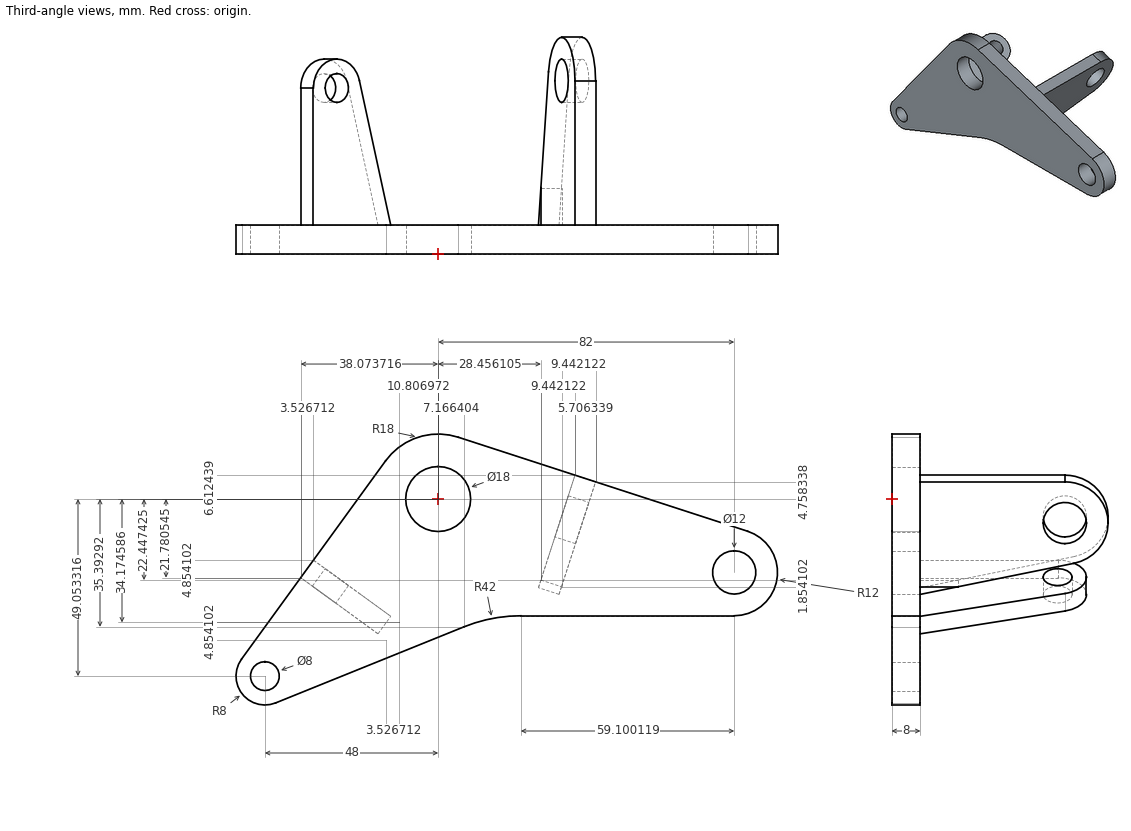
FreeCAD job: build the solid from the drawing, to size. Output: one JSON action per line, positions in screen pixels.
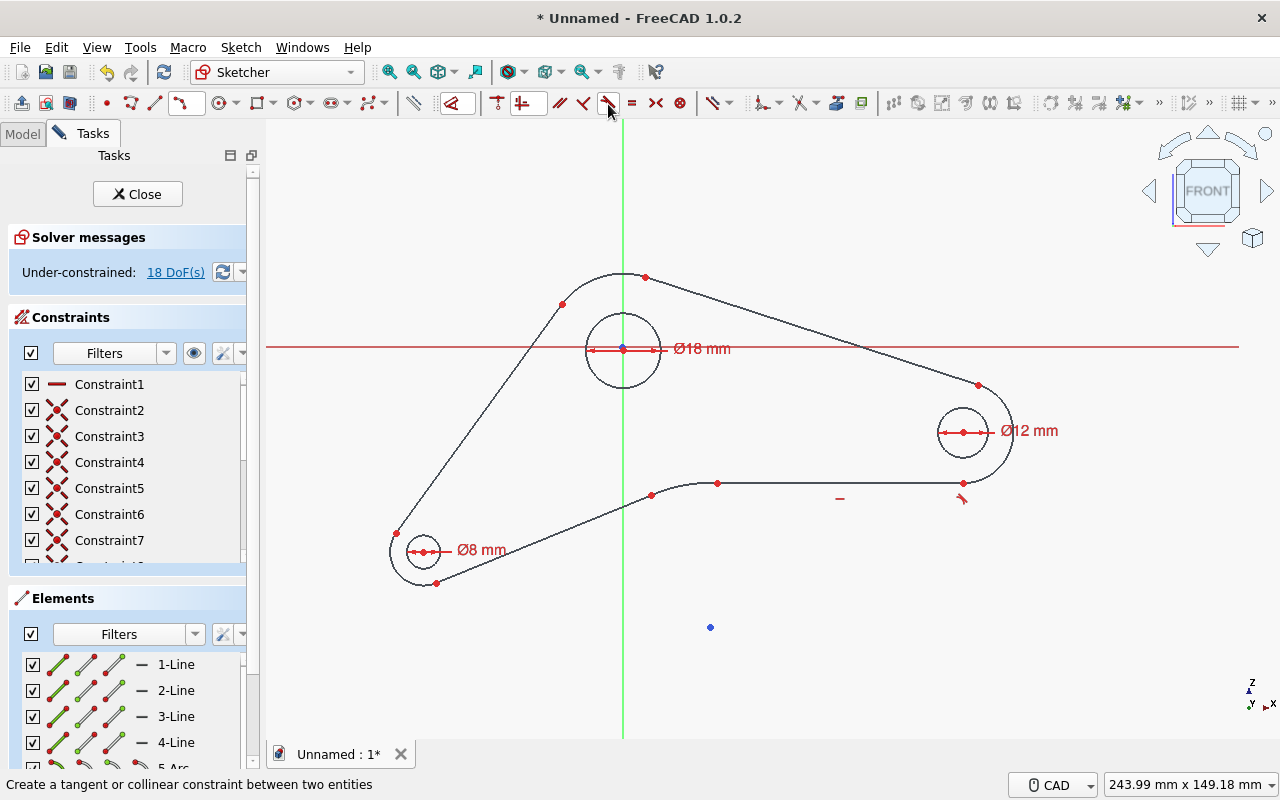
{"action": "left_click", "coordinate": [587, 522]}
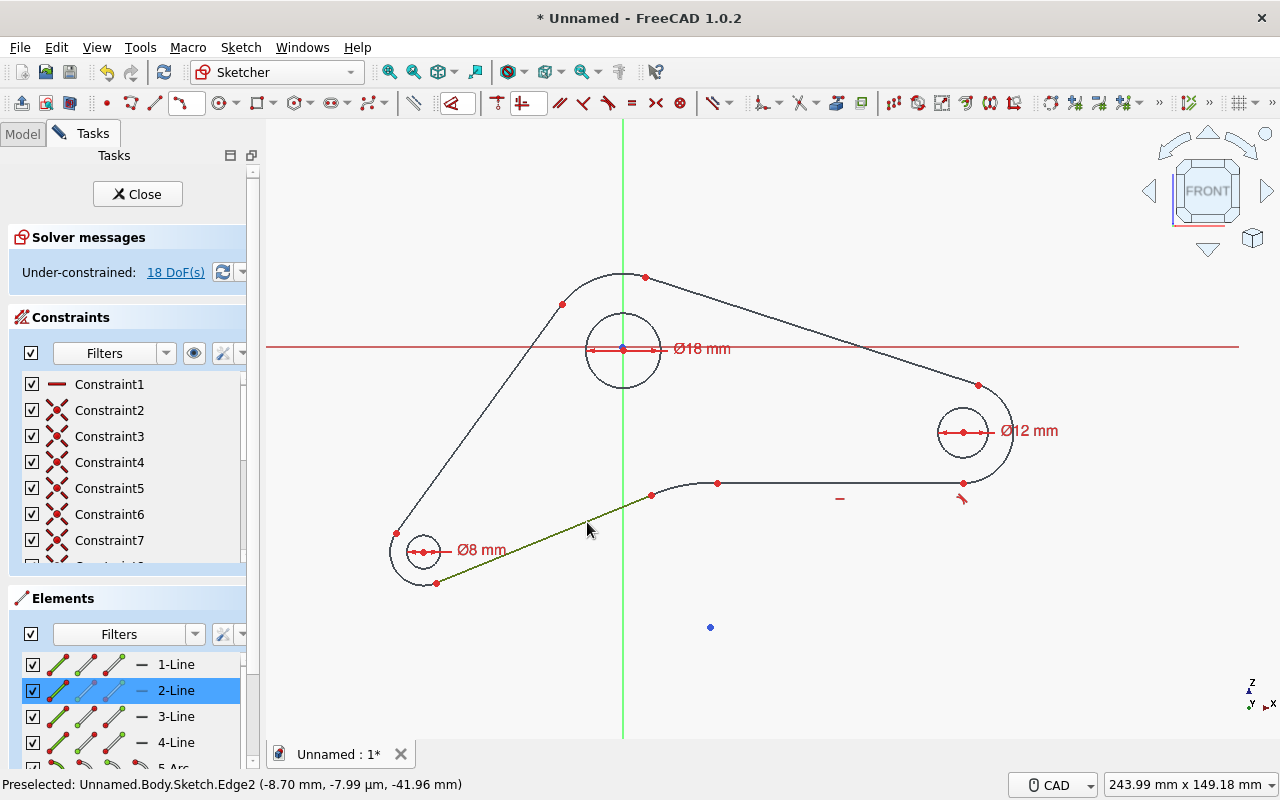
{"action": "left_click", "coordinate": [698, 483]}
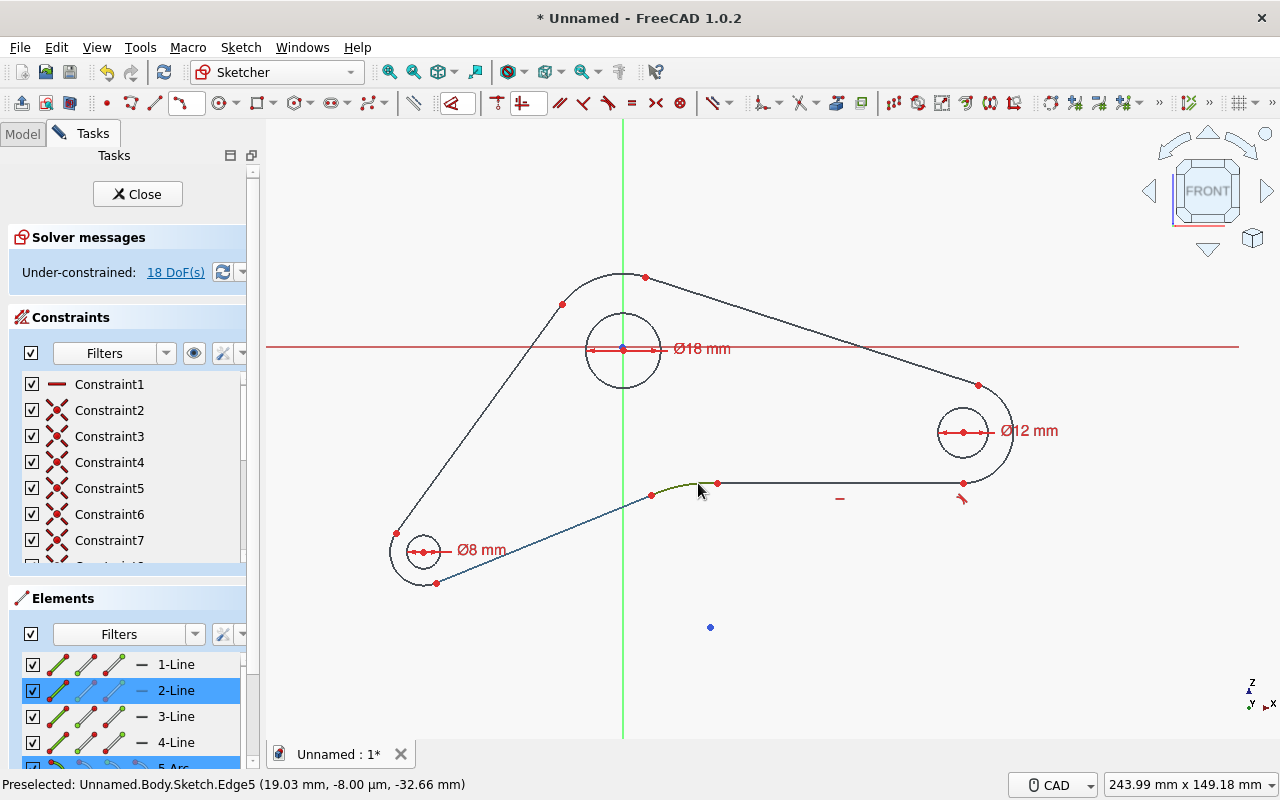
{"action": "left_click", "coordinate": [608, 104]}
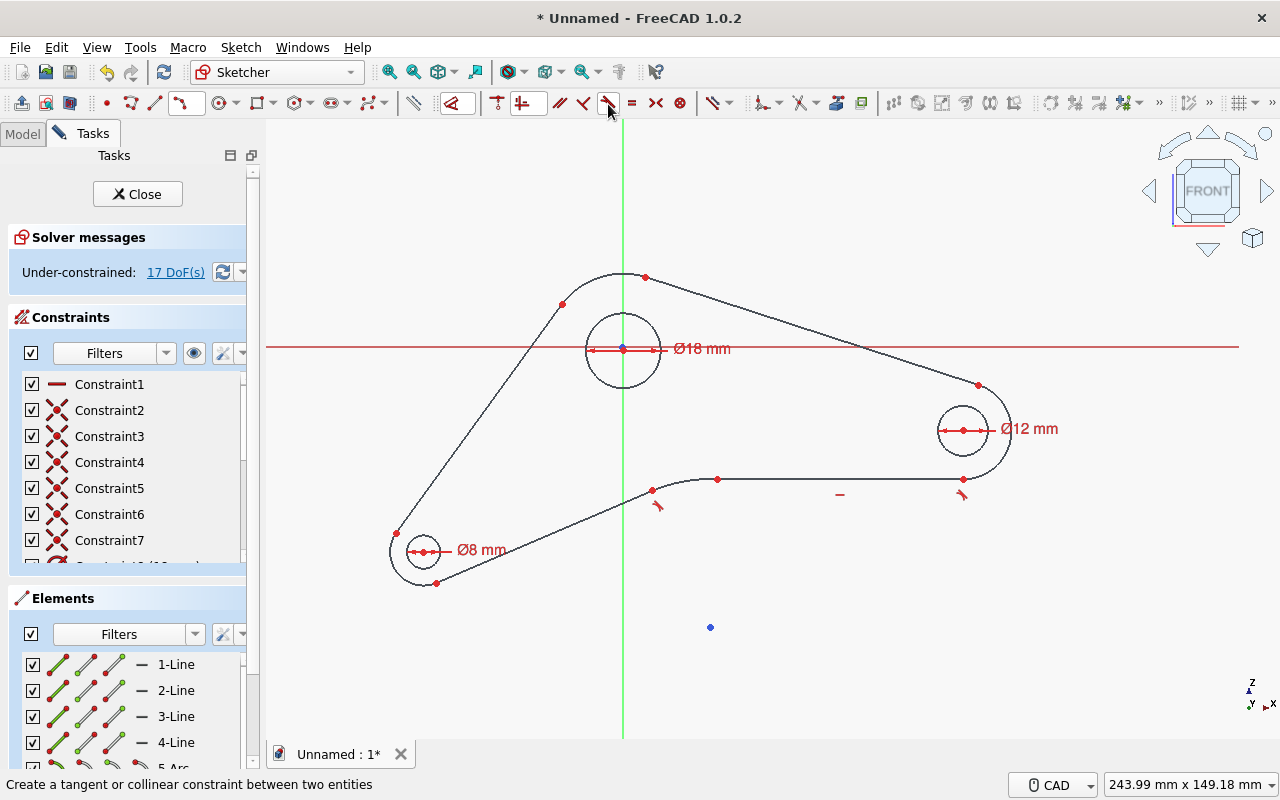
{"action": "left_click", "coordinate": [587, 519]}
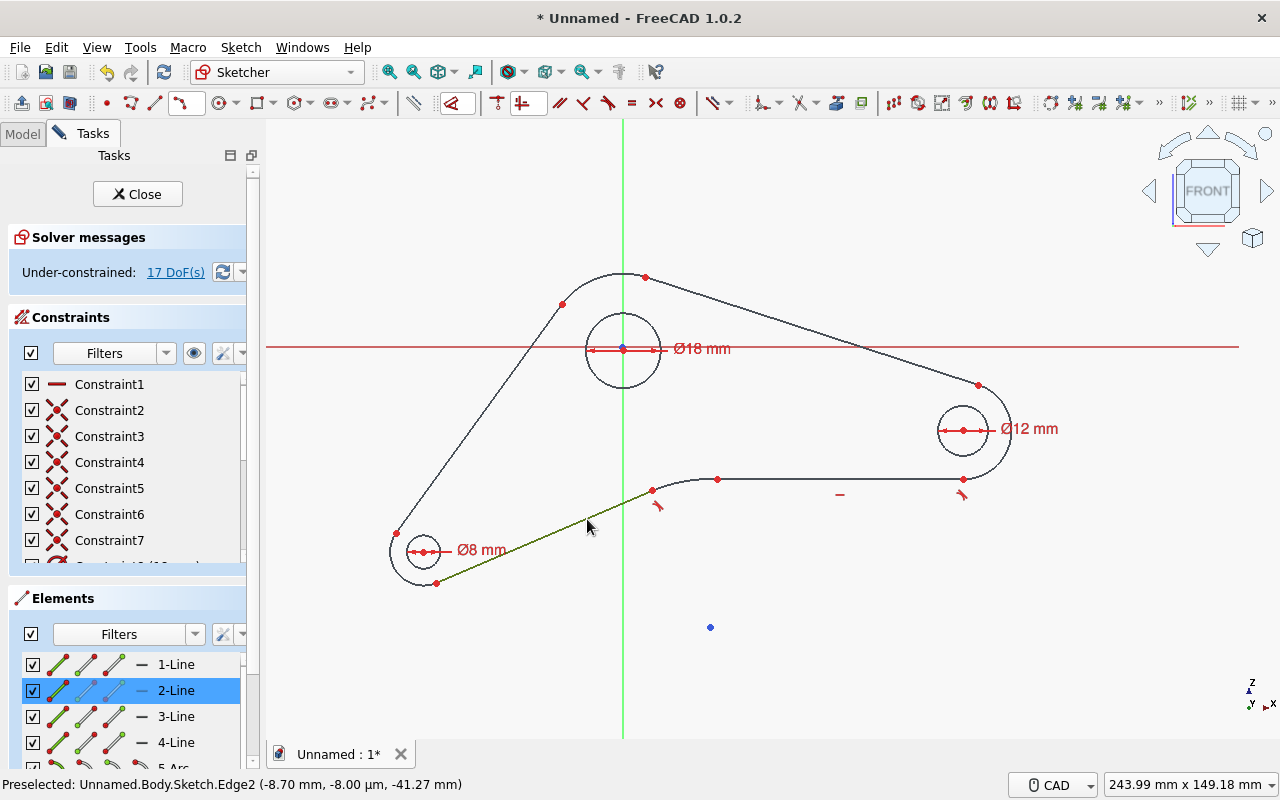
{"action": "left_click", "coordinate": [391, 558]}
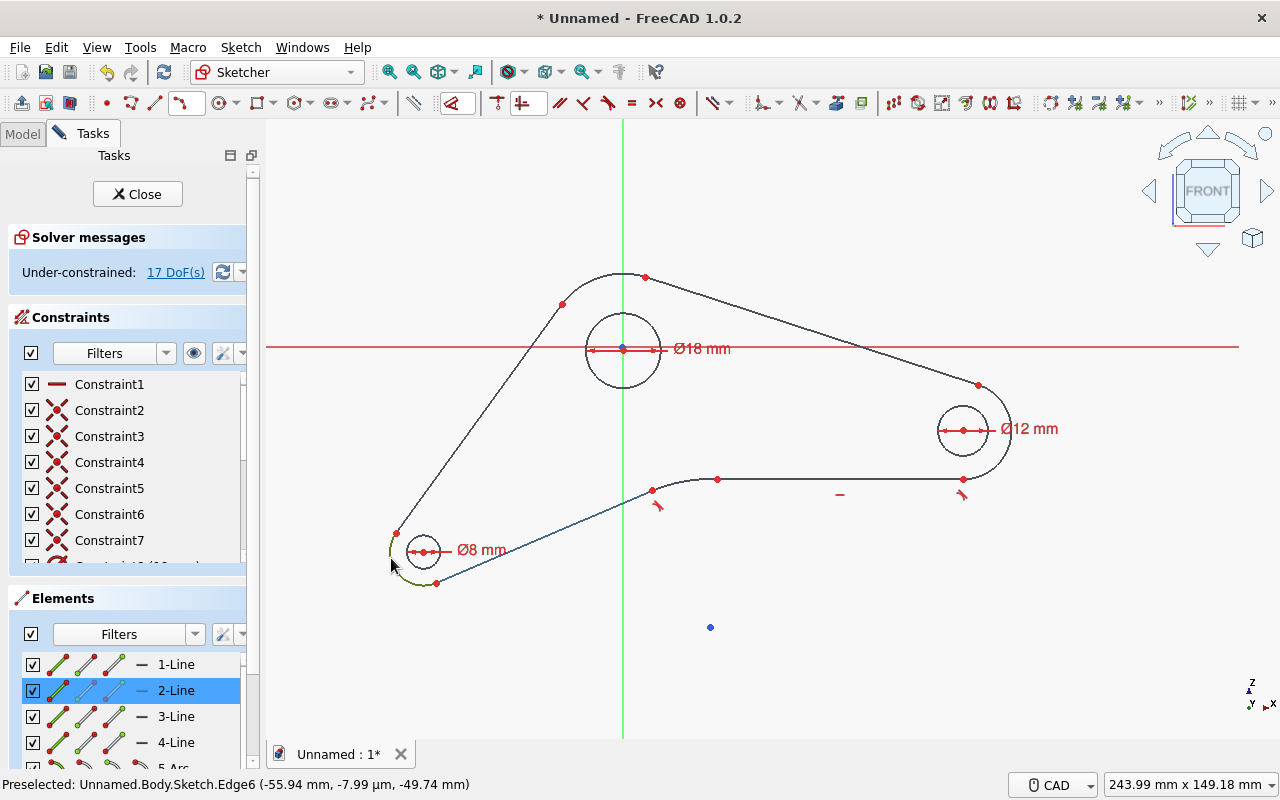
{"action": "left_click", "coordinate": [608, 104]}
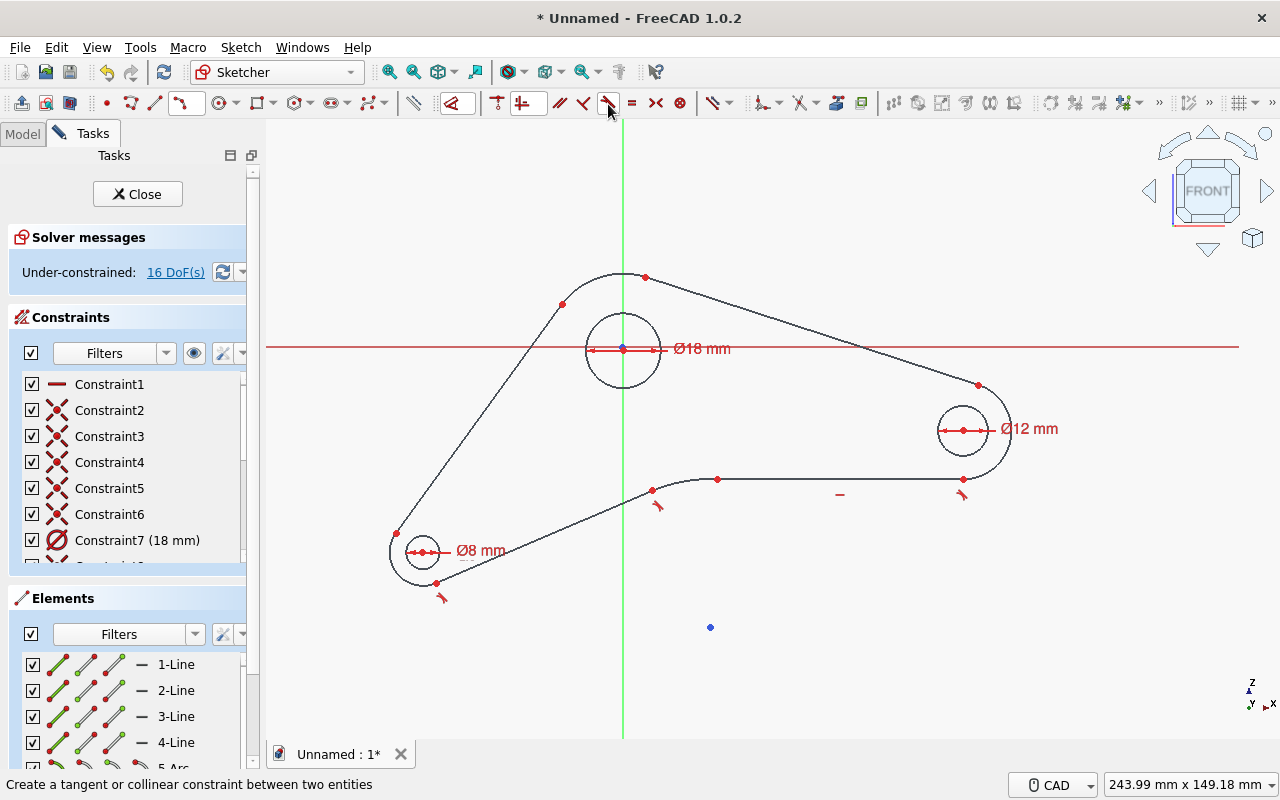
{"action": "left_click", "coordinate": [446, 464]}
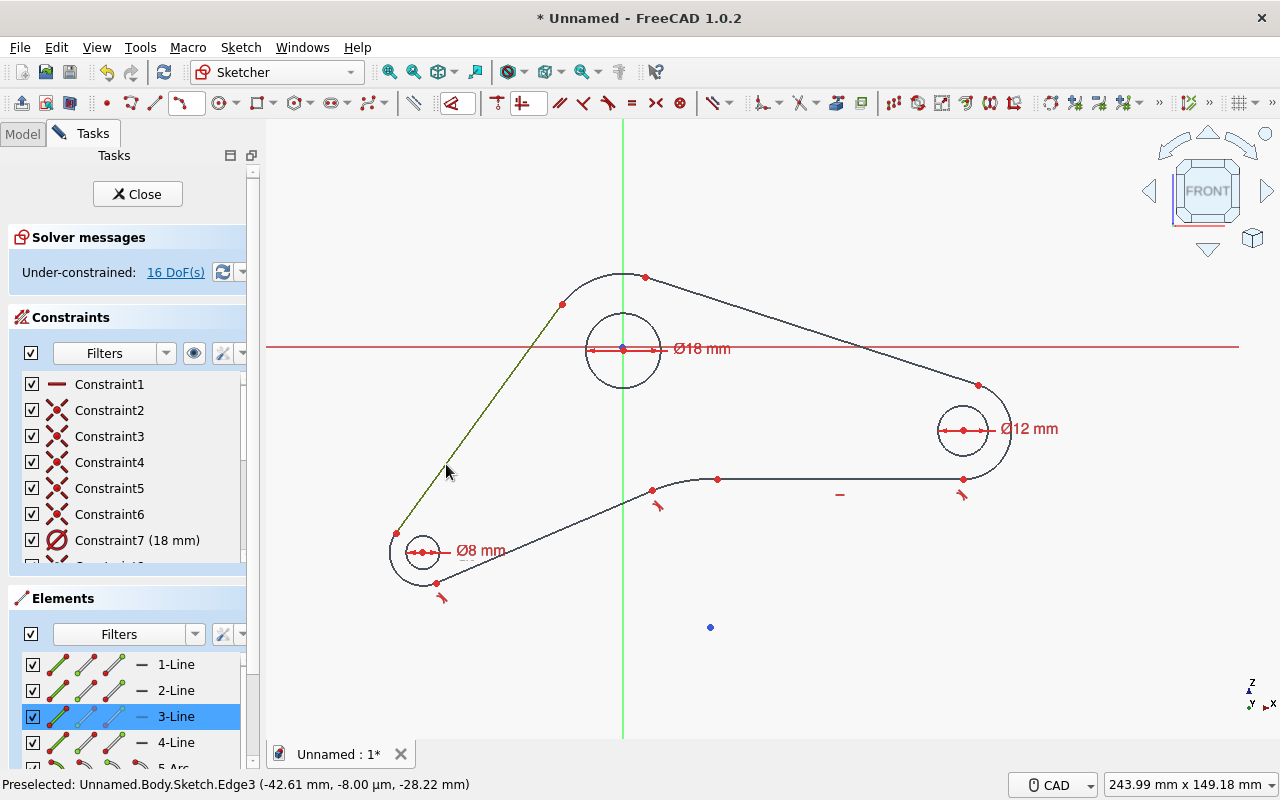
{"action": "left_click", "coordinate": [390, 558]}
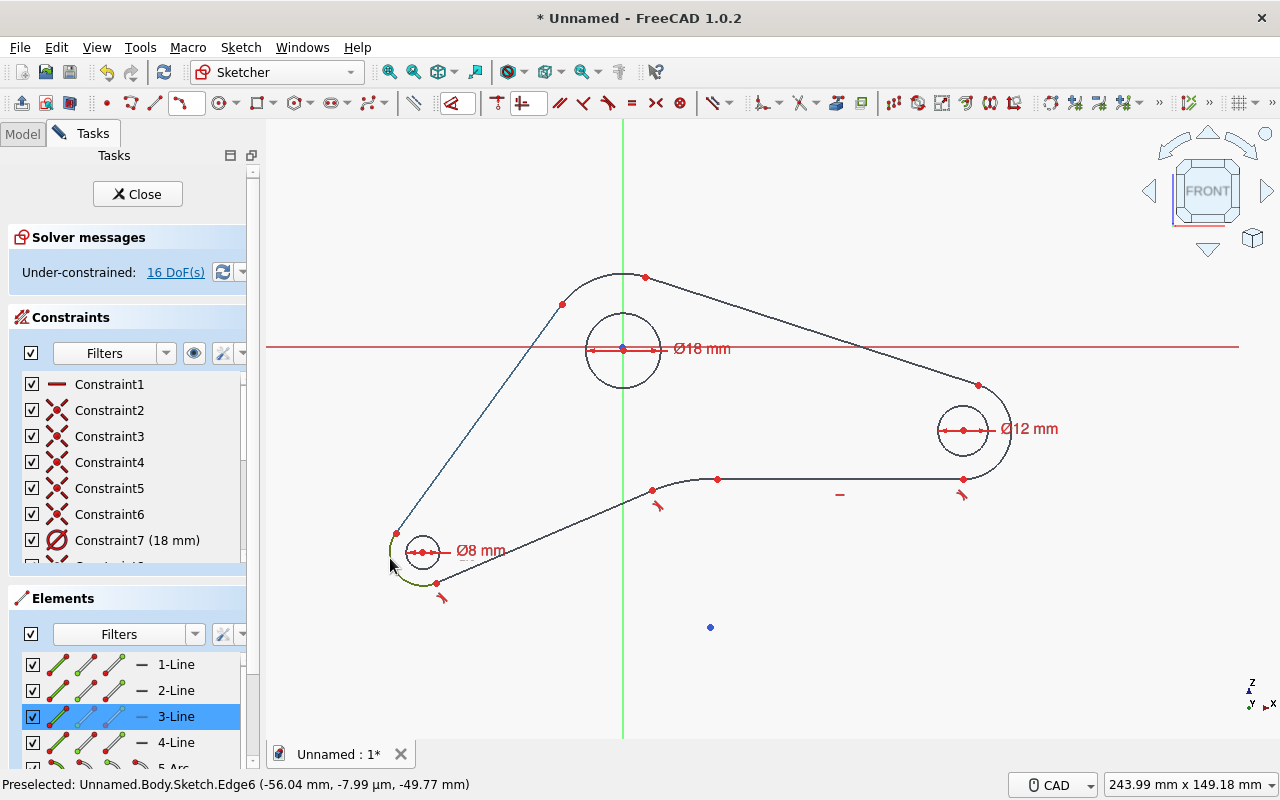
{"action": "left_click", "coordinate": [608, 104]}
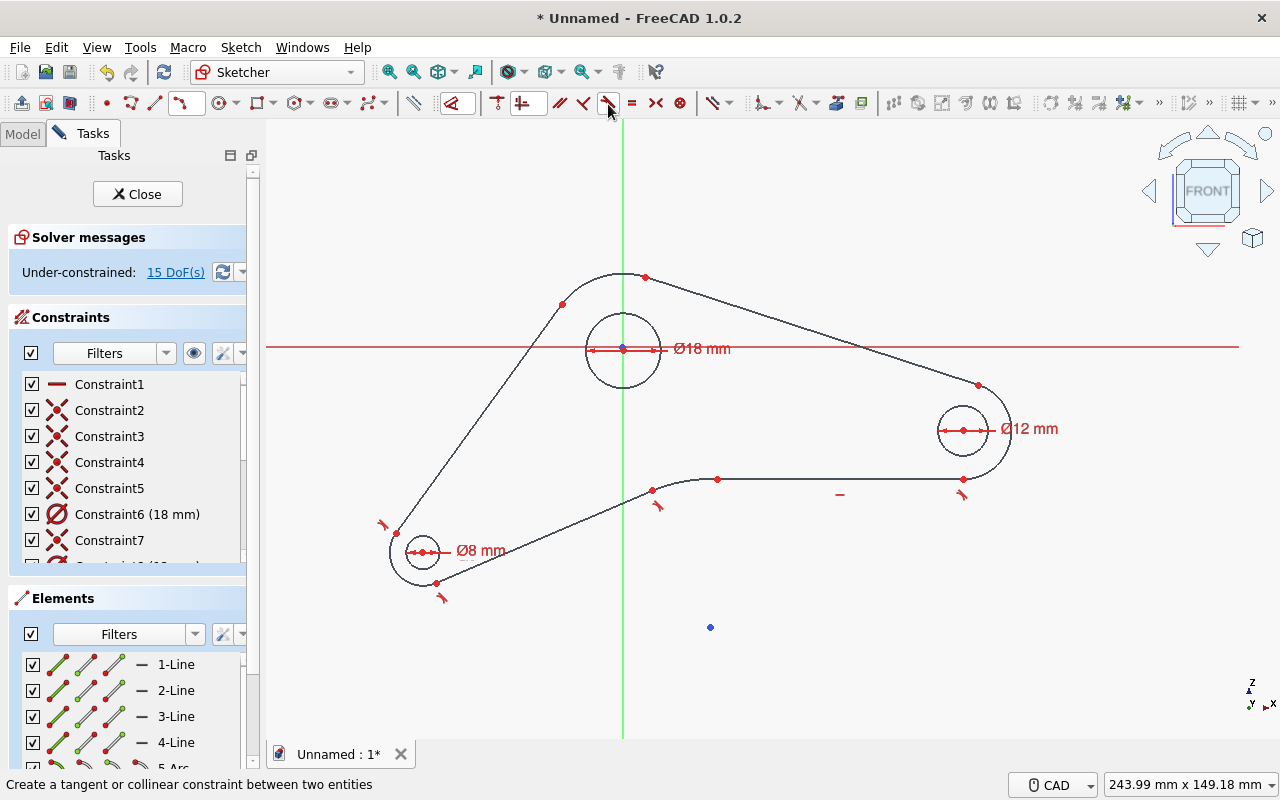
{"action": "left_click", "coordinate": [446, 464]}